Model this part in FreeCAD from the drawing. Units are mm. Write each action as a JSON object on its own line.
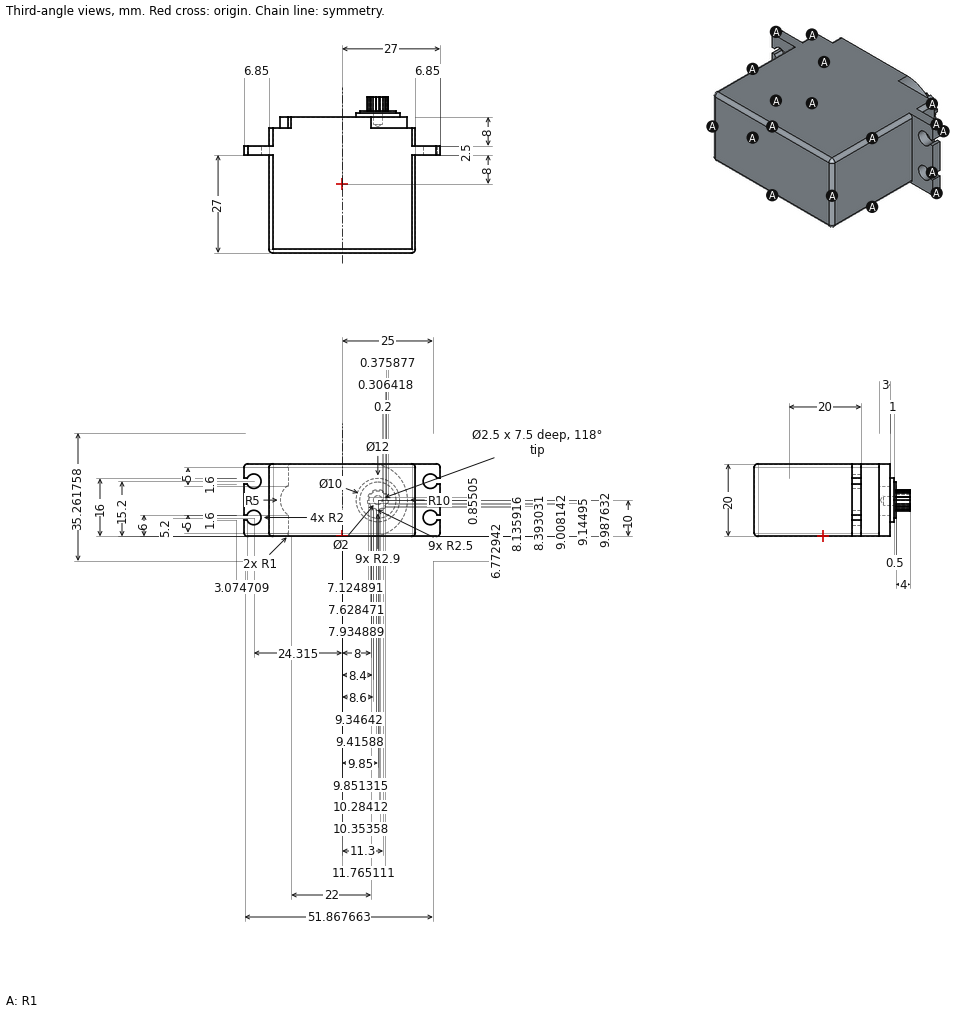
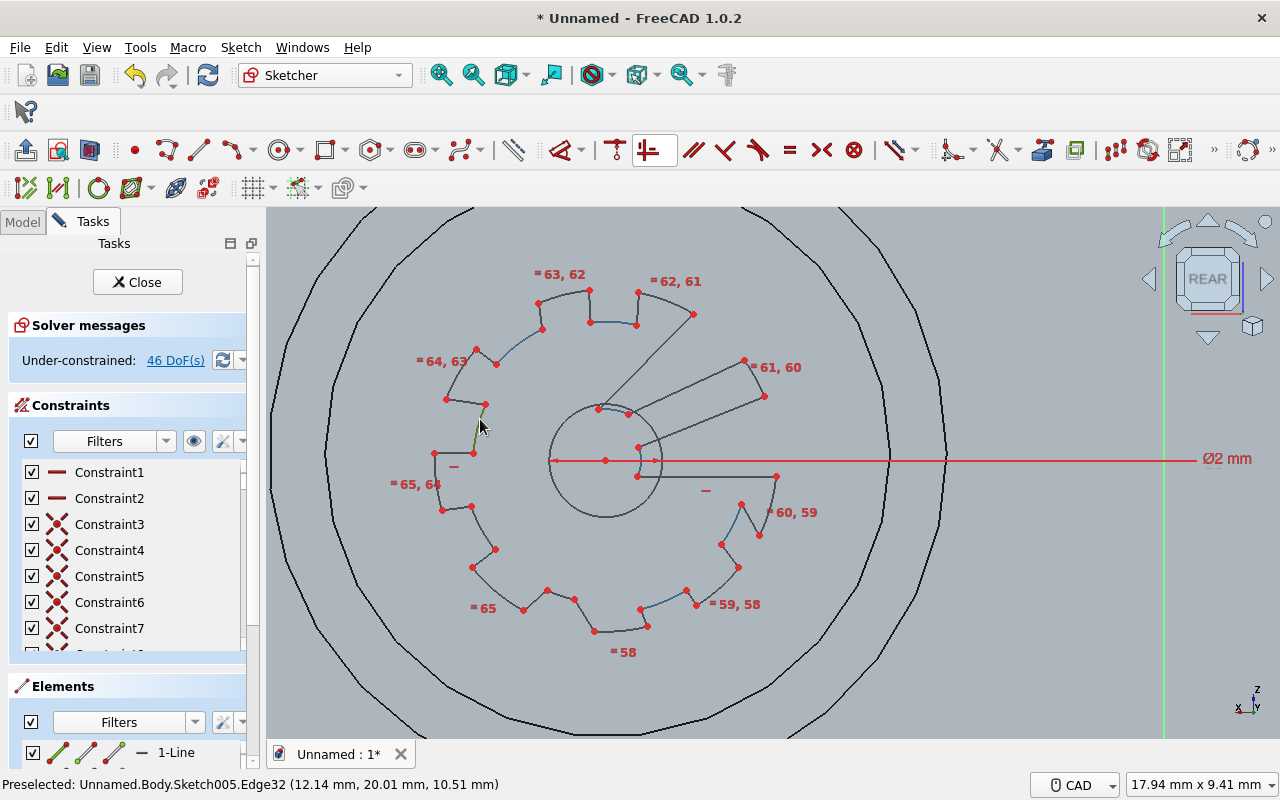
{"action": "left_click", "coordinate": [477, 520]}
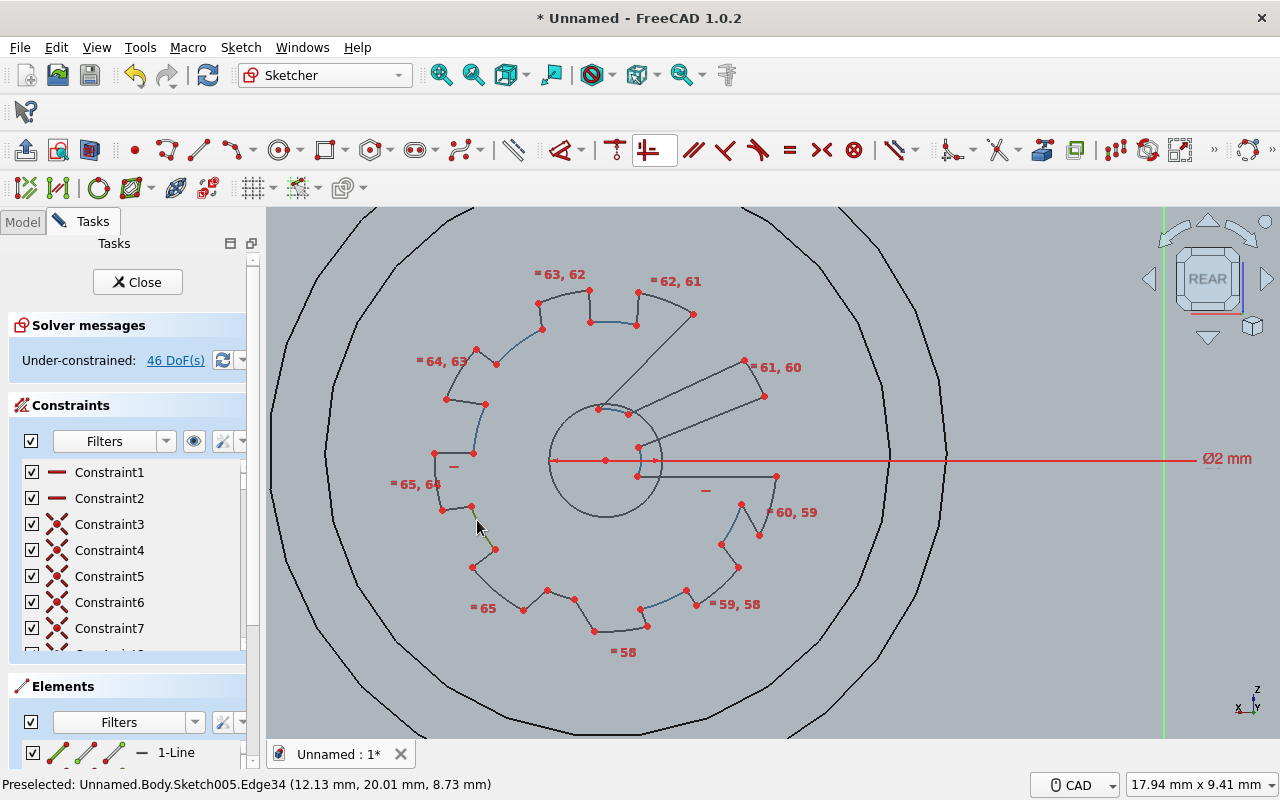
{"action": "left_click", "coordinate": [561, 596]}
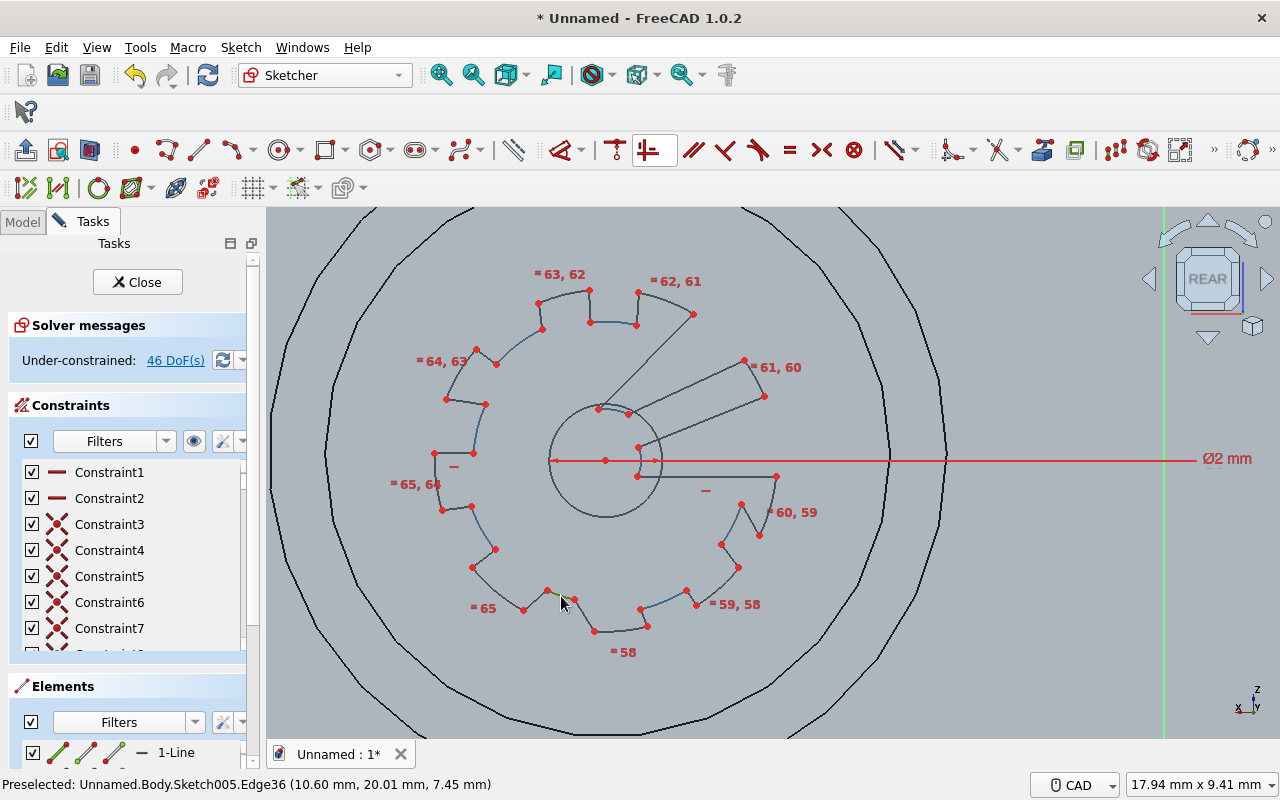
{"action": "left_click", "coordinate": [790, 150]}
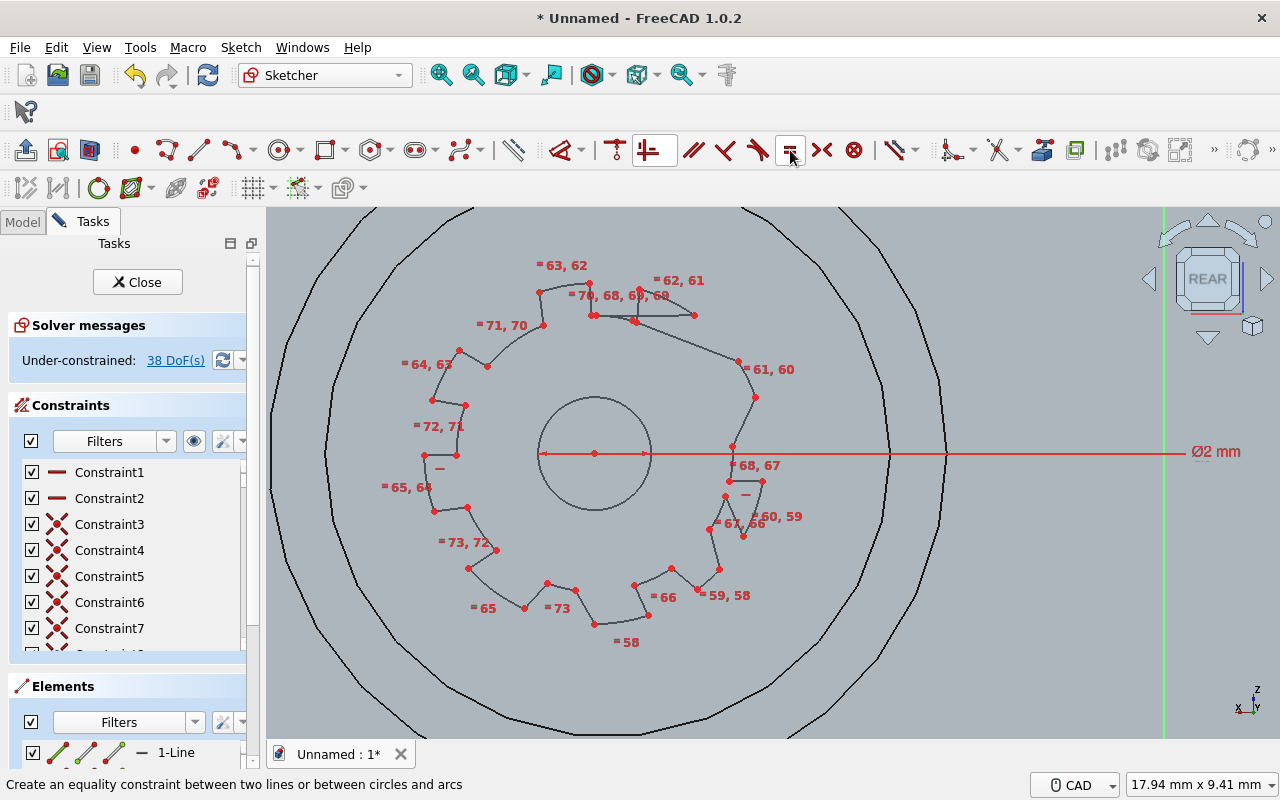
{"action": "left_click", "coordinate": [560, 150]}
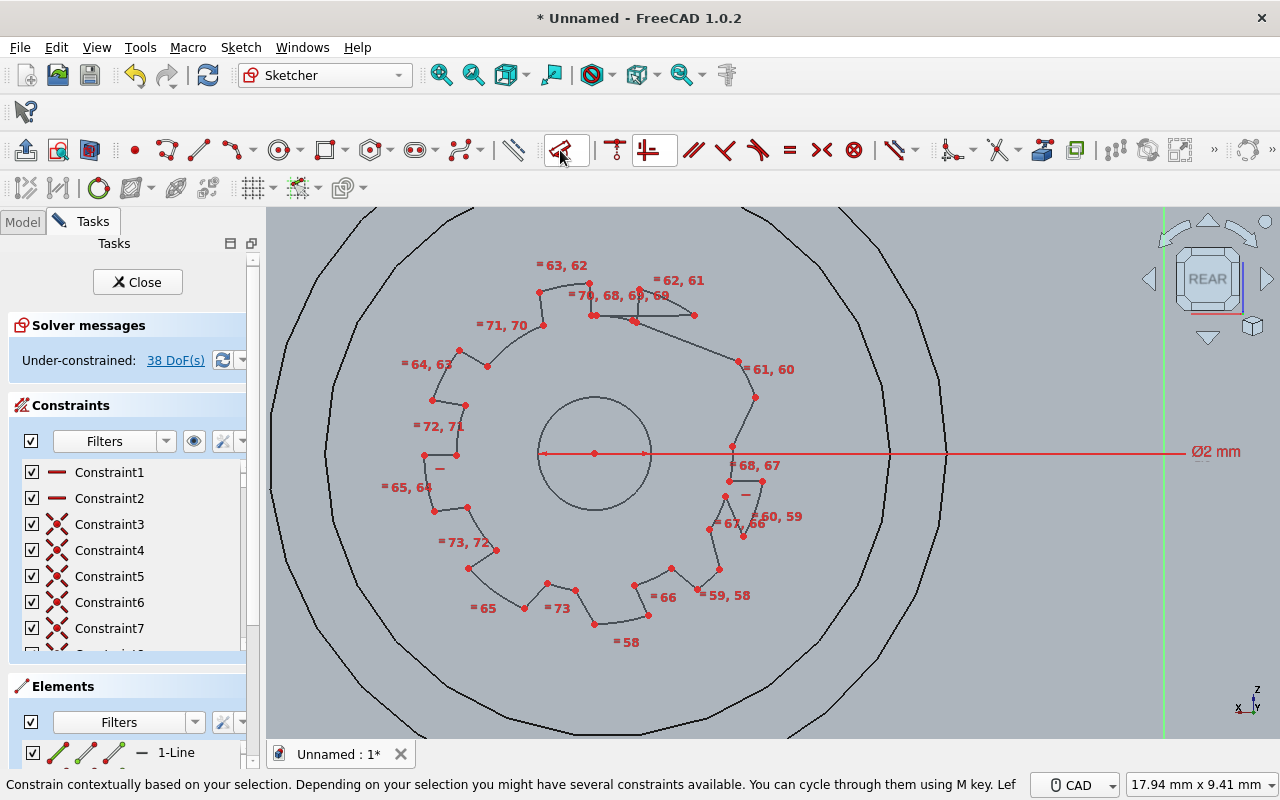
{"action": "left_click", "coordinate": [611, 623]}
{"action": "left_click", "coordinate": [614, 655]}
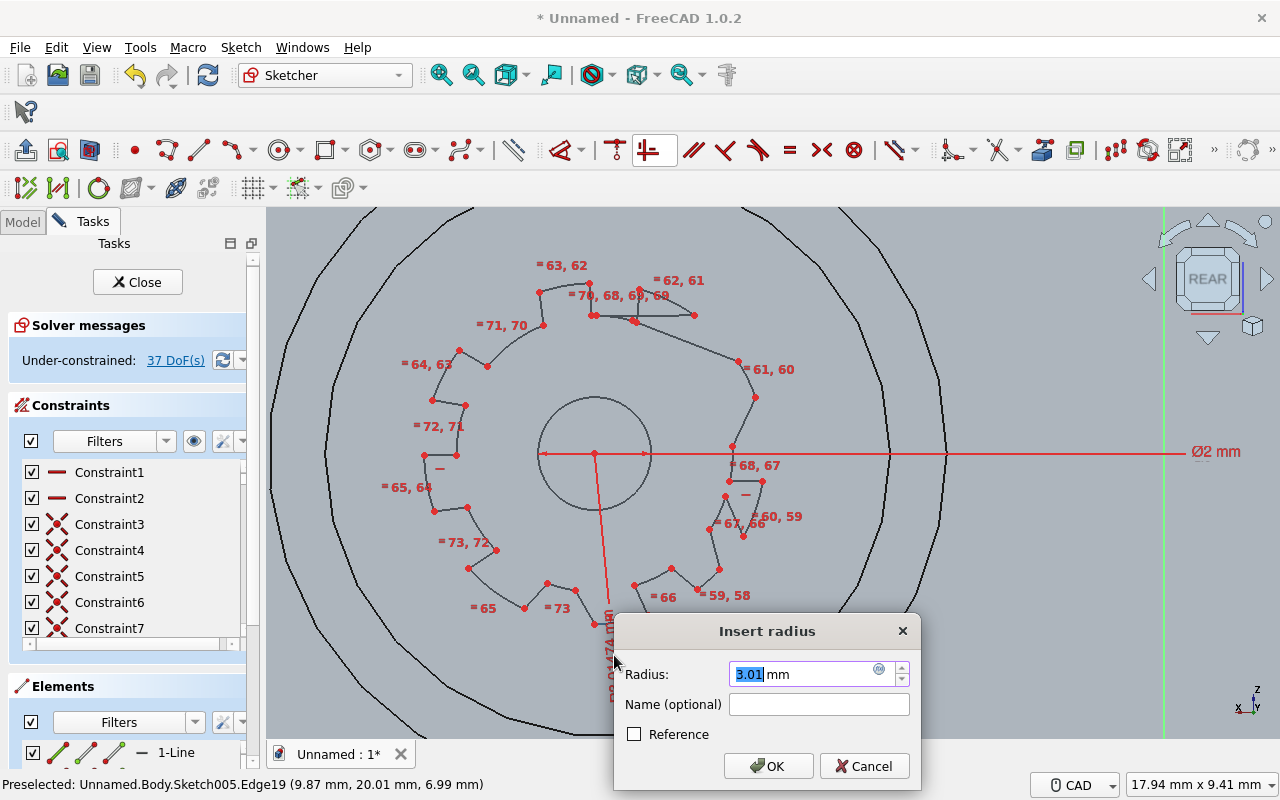
{"action": "type", "text": "2.9"}
{"action": "key", "text": "Return"}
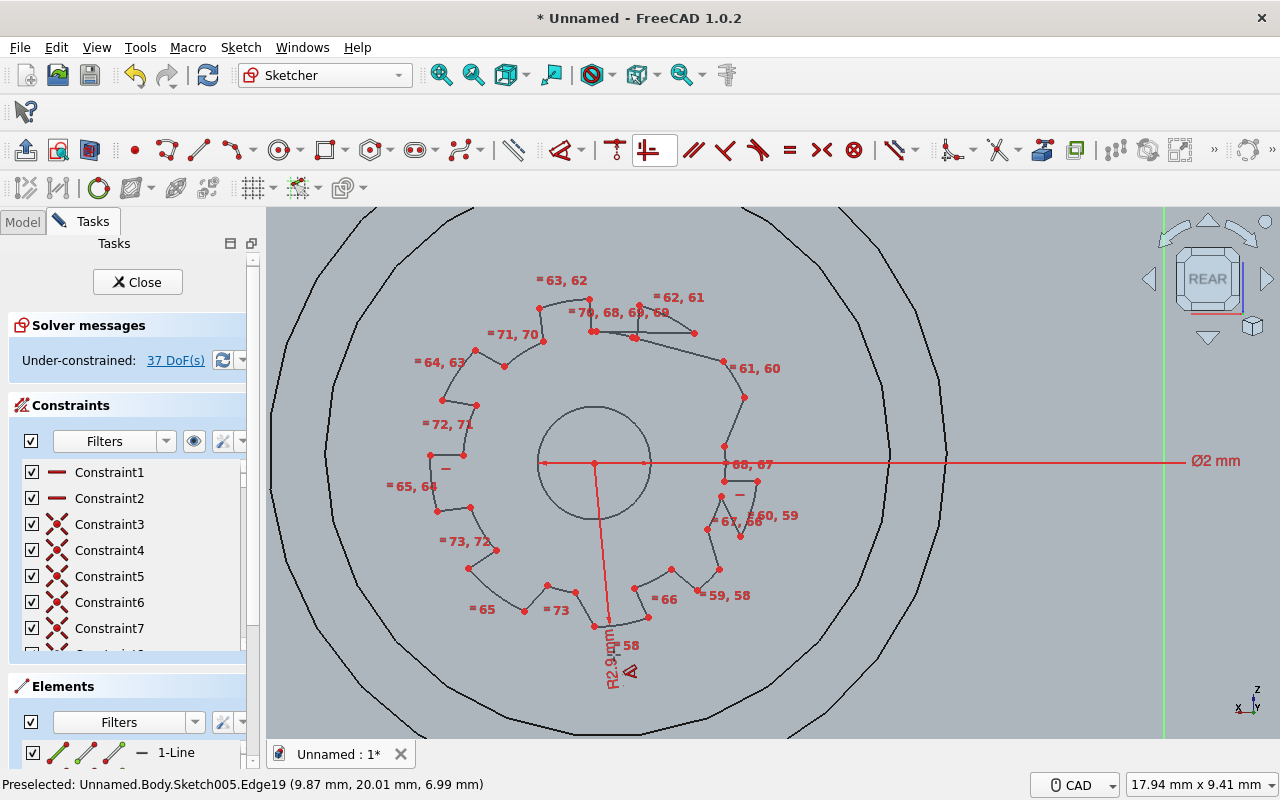
{"action": "left_click", "coordinate": [646, 584]}
{"action": "left_click", "coordinate": [579, 626]}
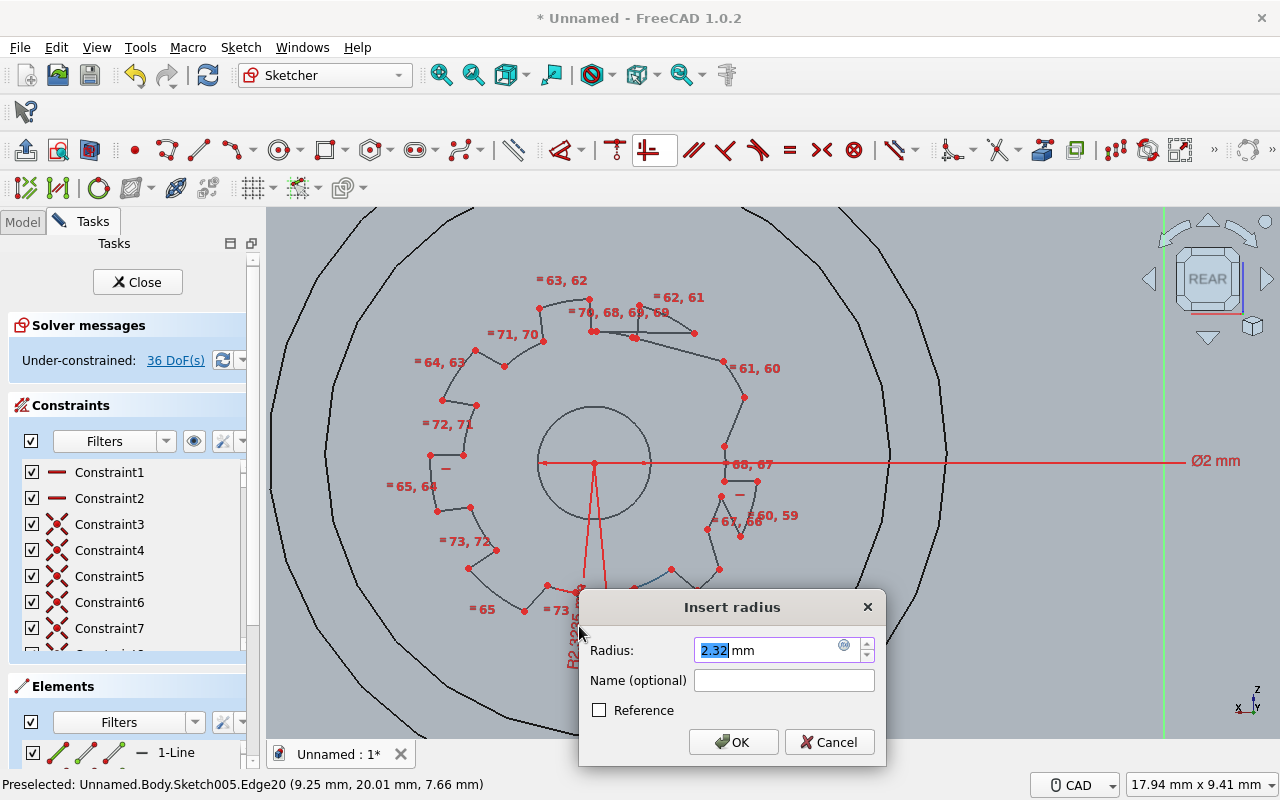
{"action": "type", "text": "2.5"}
{"action": "key", "text": "Return"}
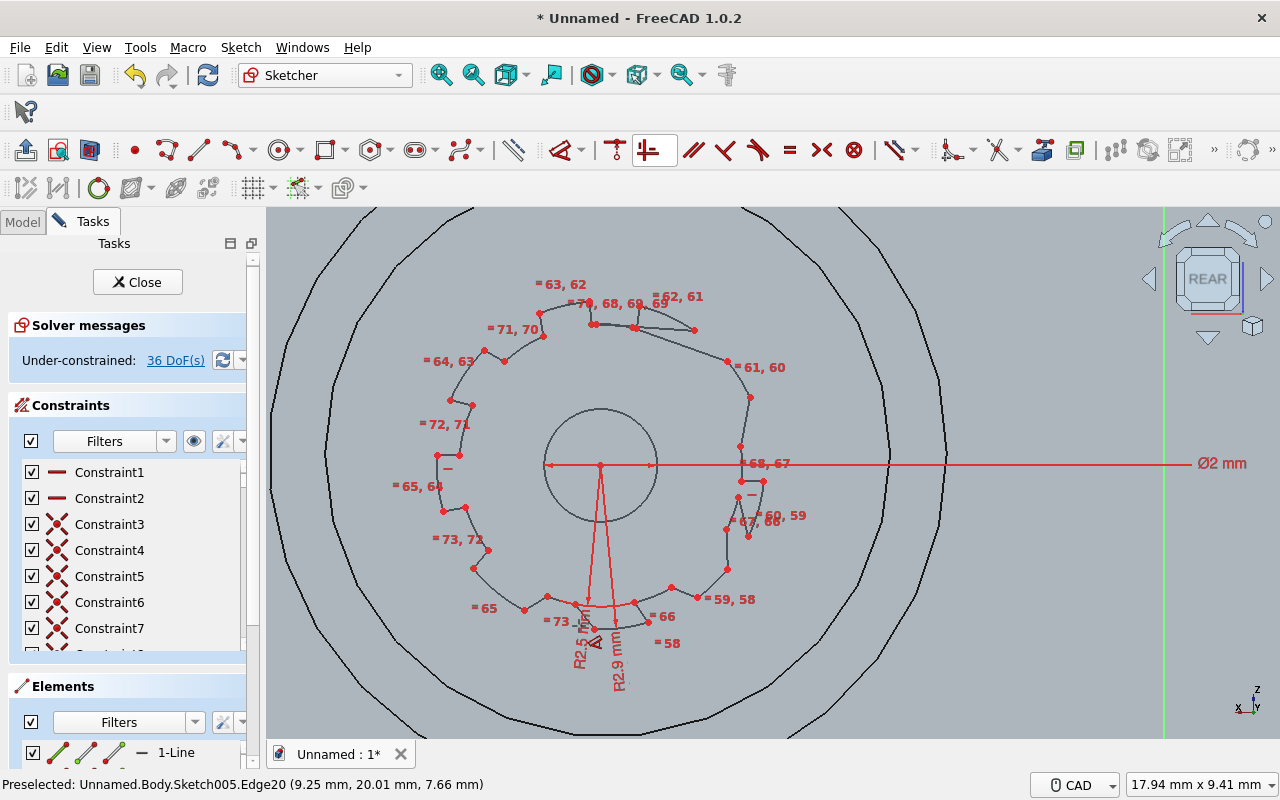
{"action": "left_click", "coordinate": [601, 465]}
{"action": "left_click", "coordinate": [567, 588]}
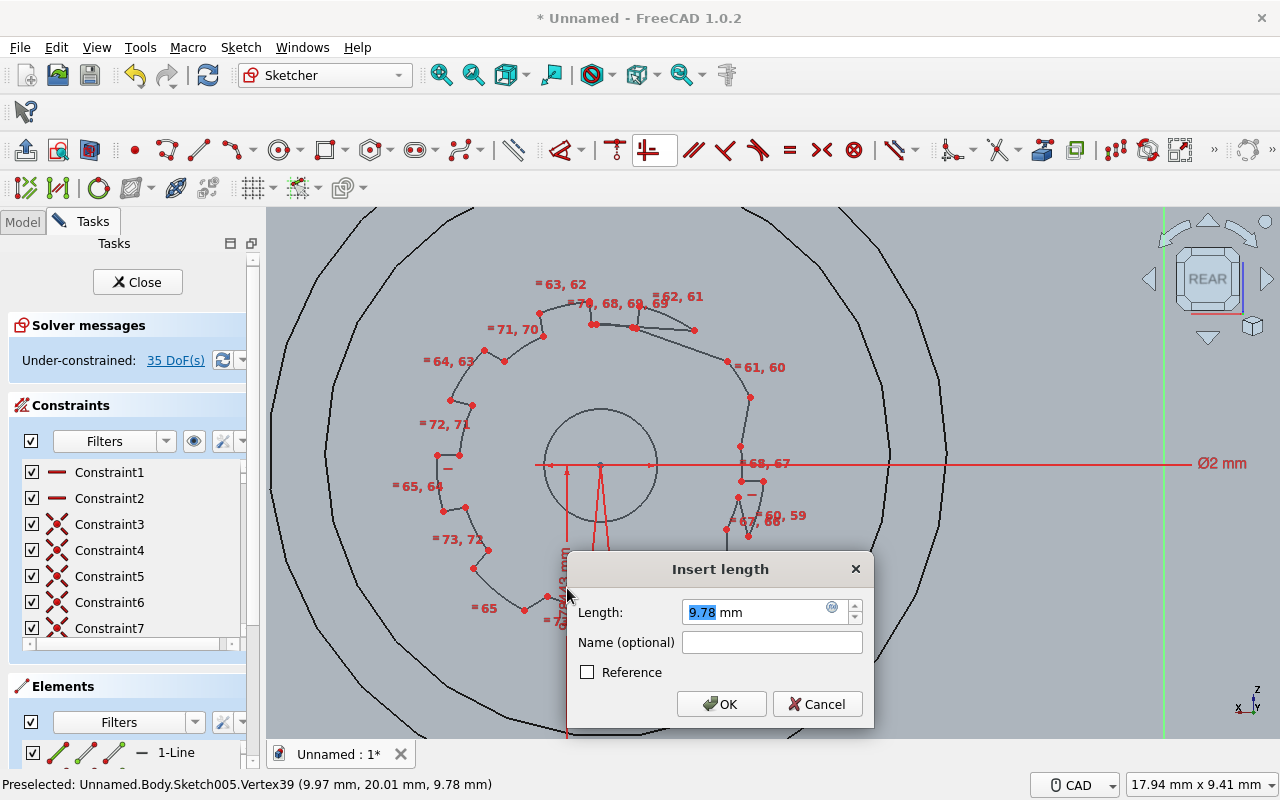
{"action": "type", "text": "10"}
{"action": "key", "text": "Return"}